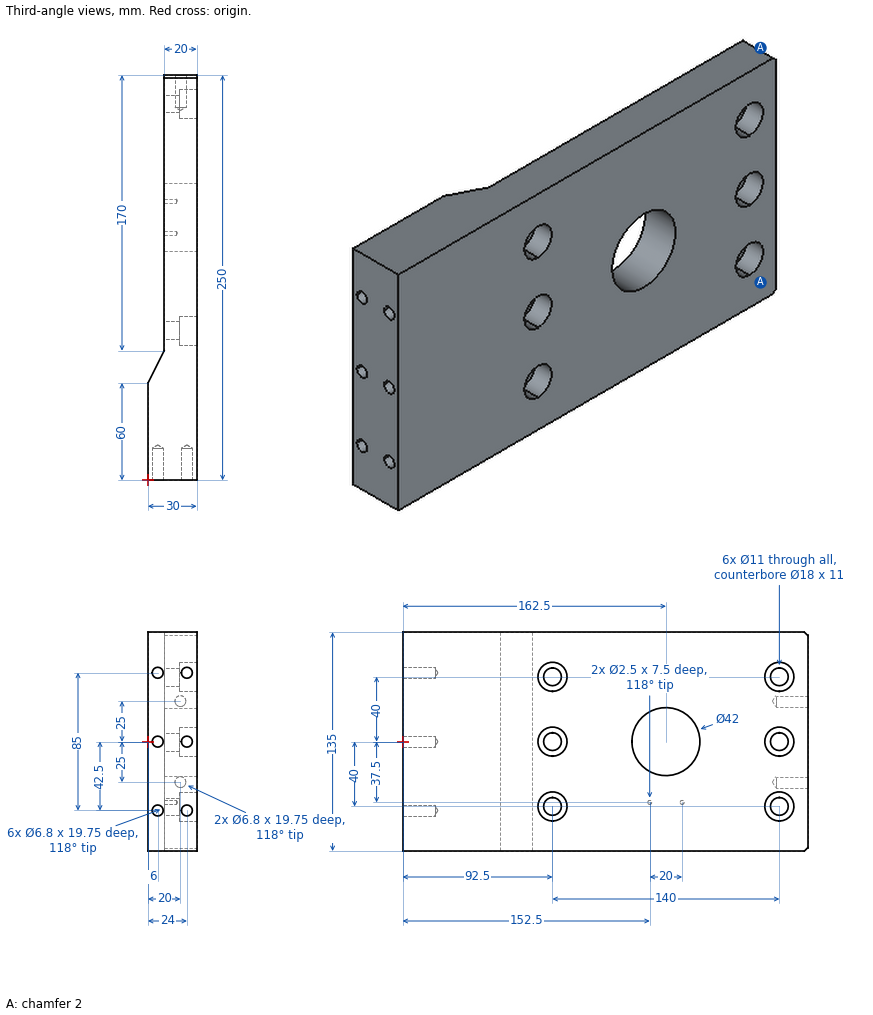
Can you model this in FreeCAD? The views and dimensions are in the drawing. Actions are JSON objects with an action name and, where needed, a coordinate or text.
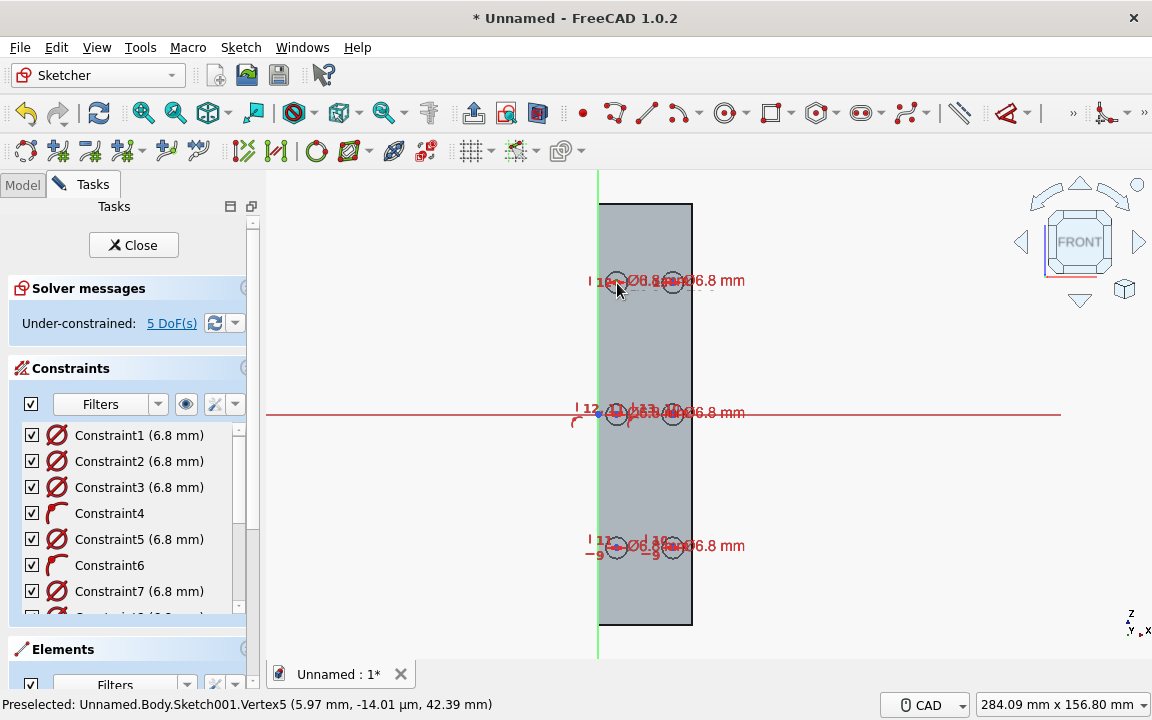
{"action": "left_click", "coordinate": [673, 283]}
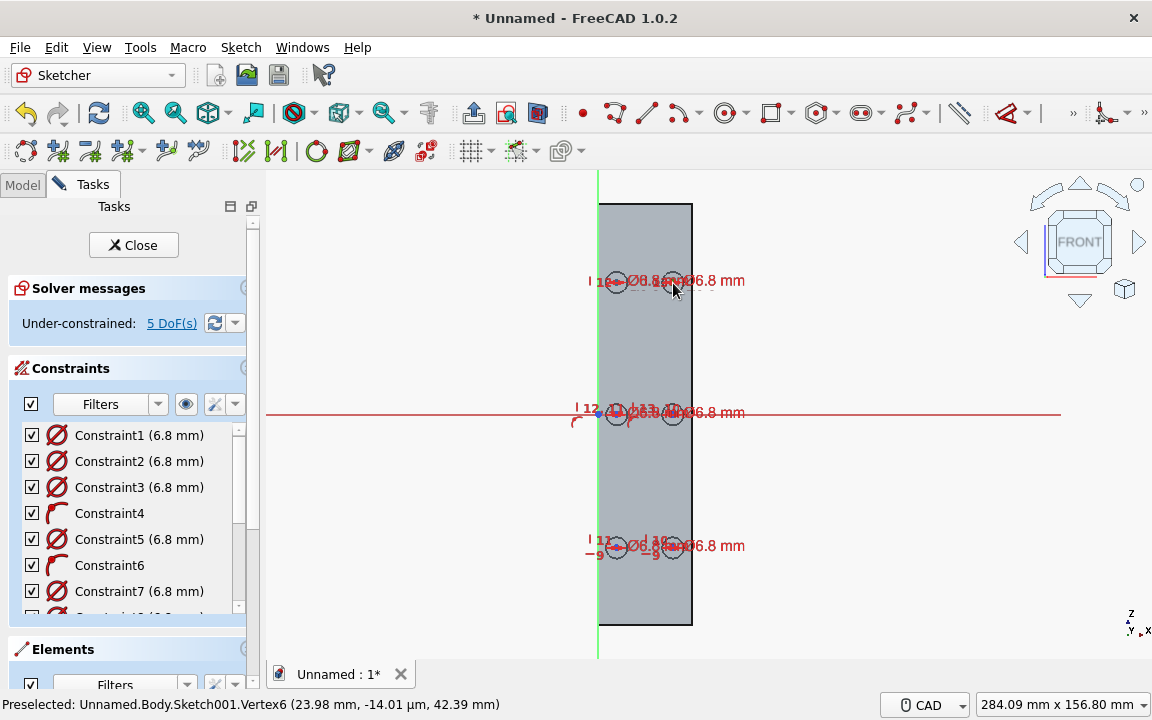
{"action": "key", "text": "h"}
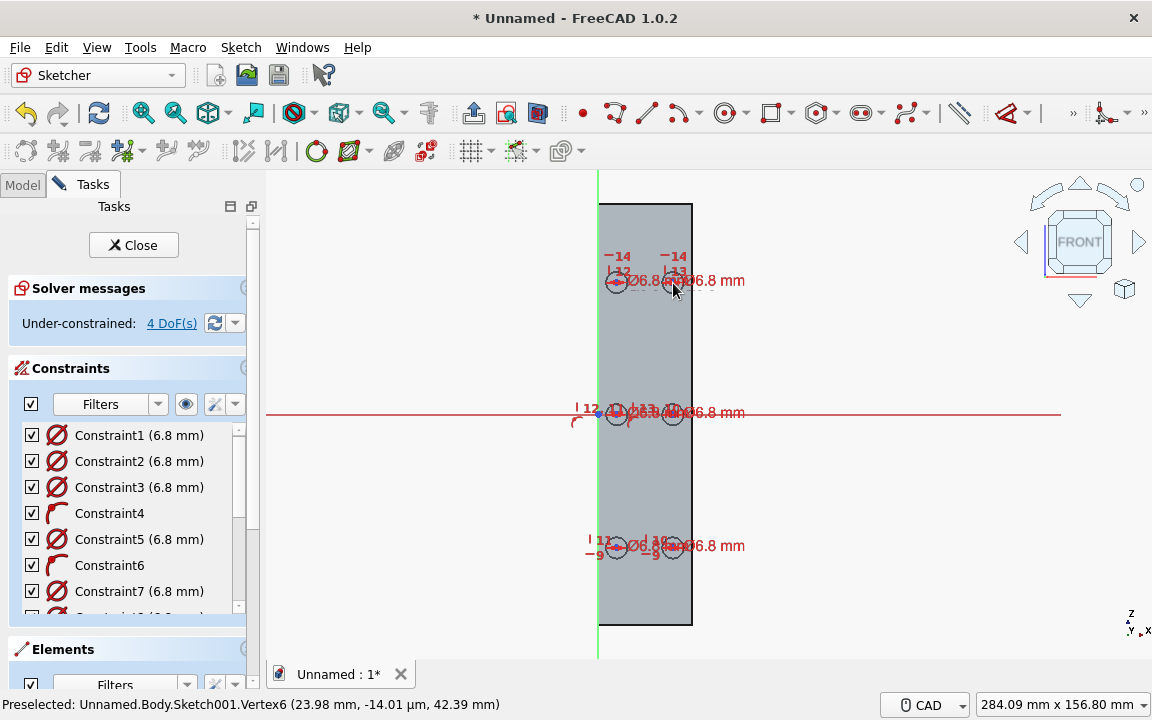
{"action": "left_click", "coordinate": [1006, 114]}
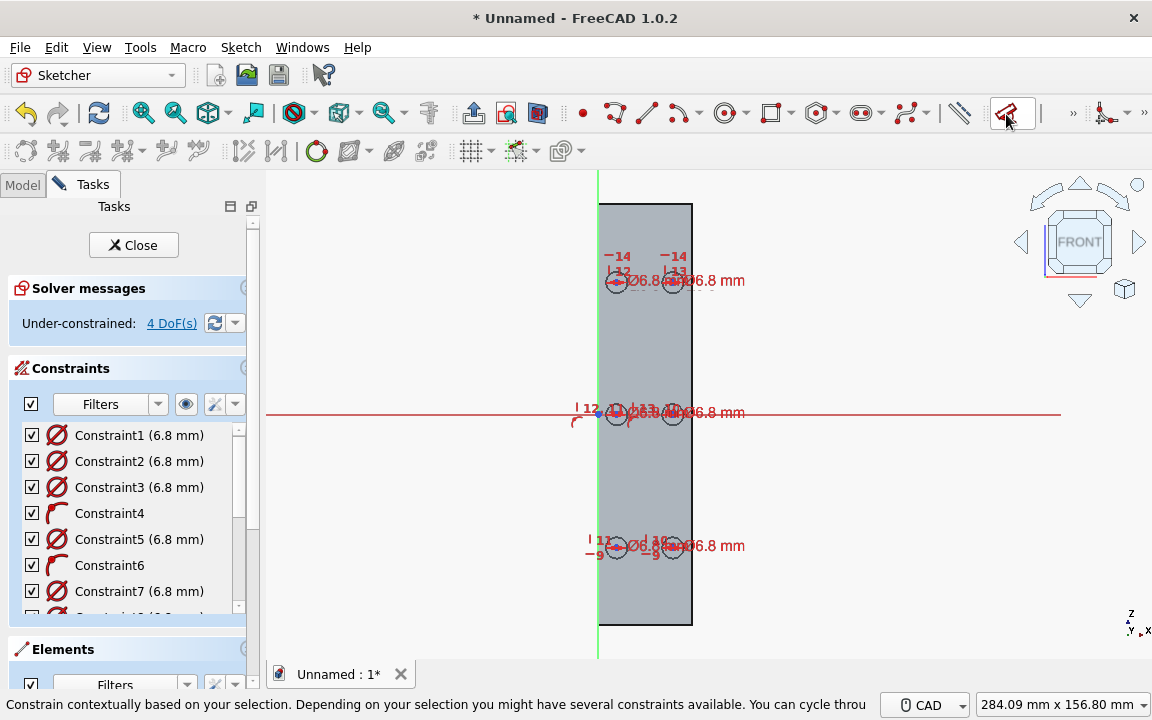
{"action": "scroll", "coordinate": [617, 548], "scroll_direction": "up", "scroll_amount": 4}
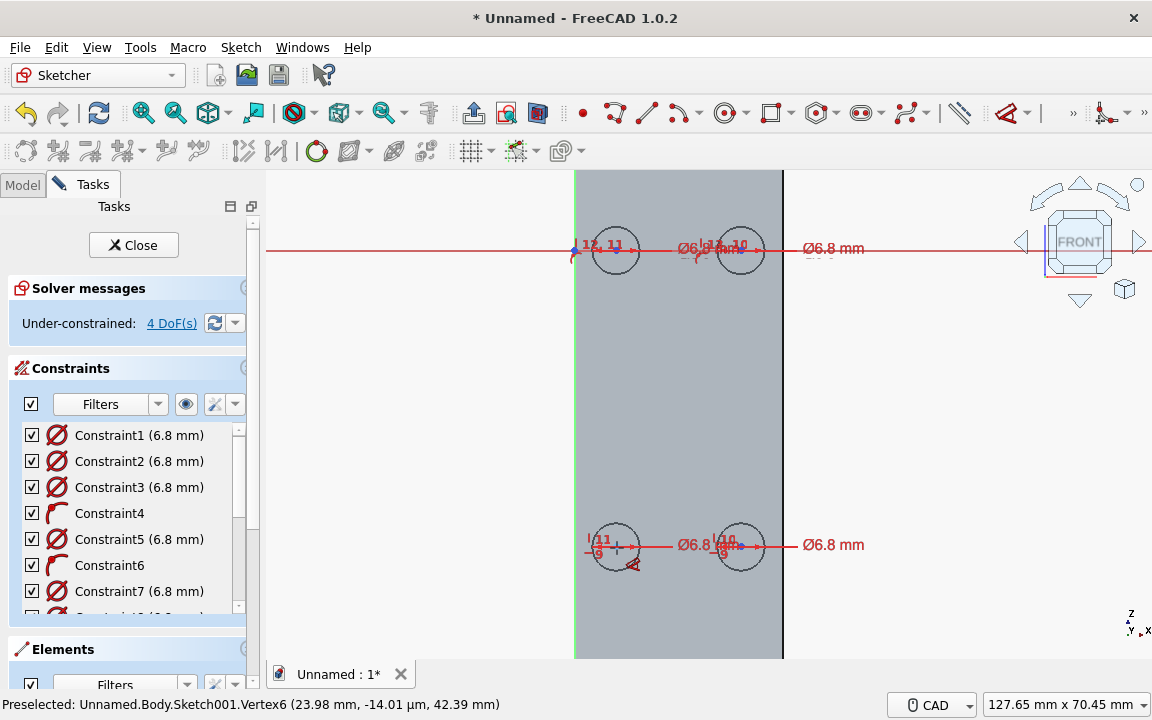
{"action": "left_click", "coordinate": [616, 547]}
{"action": "left_click", "coordinate": [595, 581]}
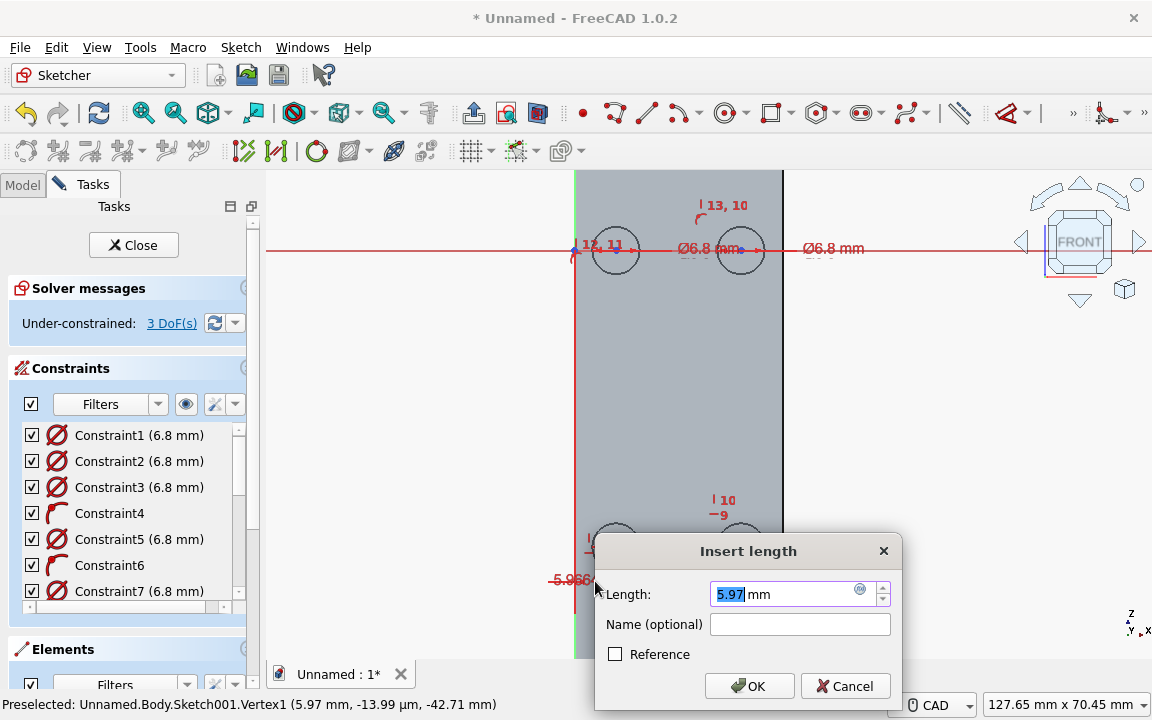
{"action": "type", "text": "6"}
{"action": "key", "text": "Return"}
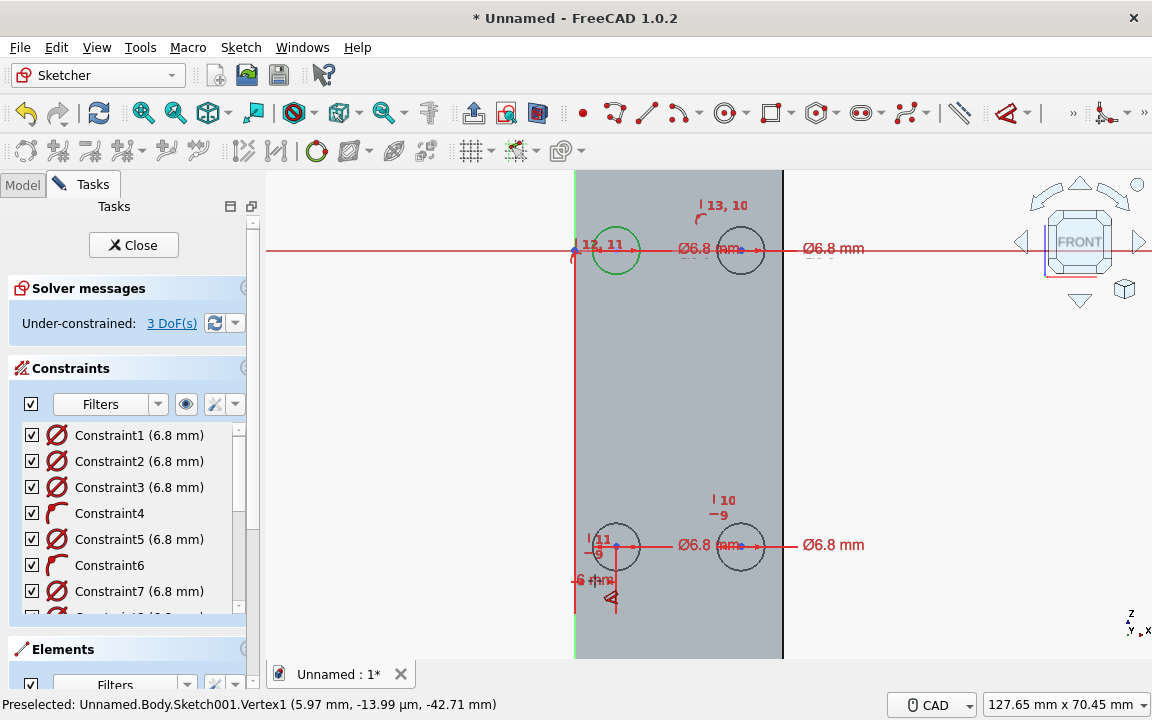
{"action": "left_click", "coordinate": [741, 547]}
{"action": "left_click", "coordinate": [696, 581]}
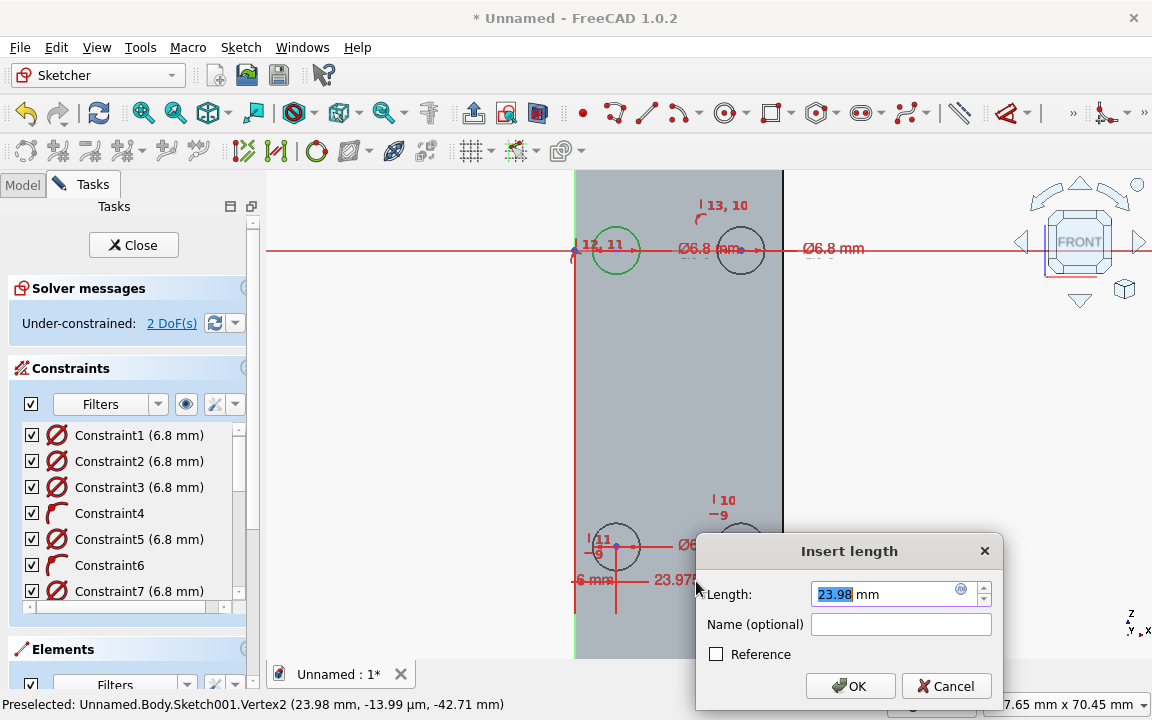
{"action": "type", "text": "24"}
{"action": "key", "text": "Return"}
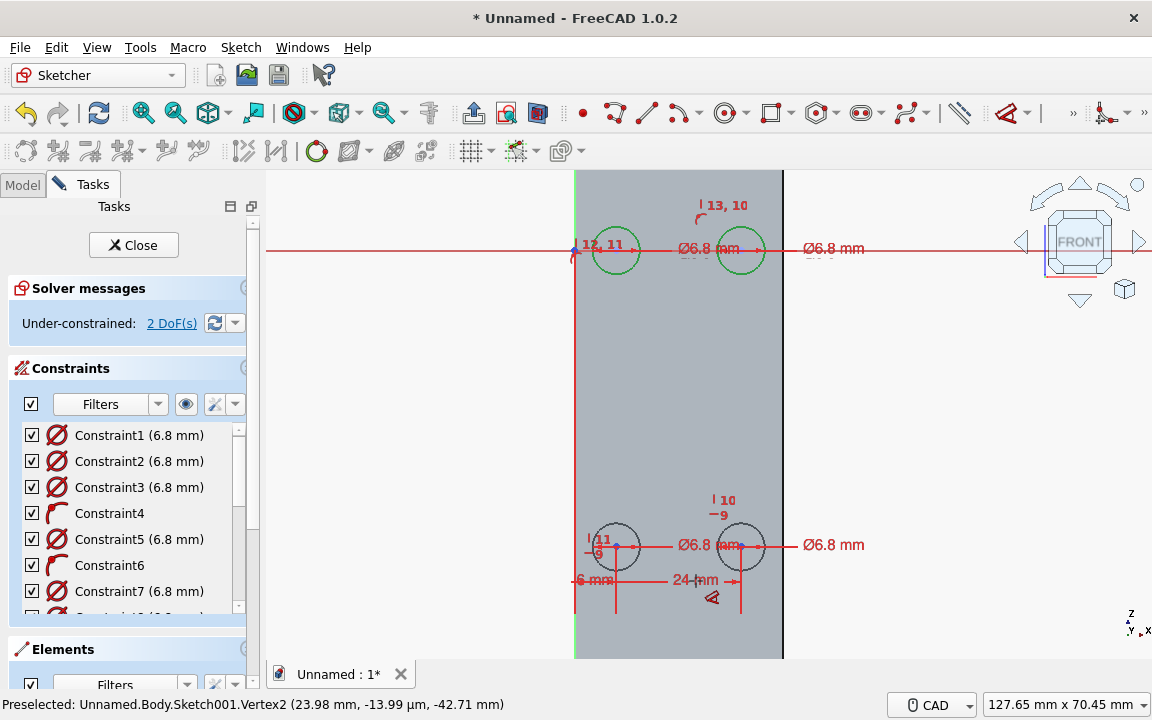
{"action": "left_click", "coordinate": [616, 547]}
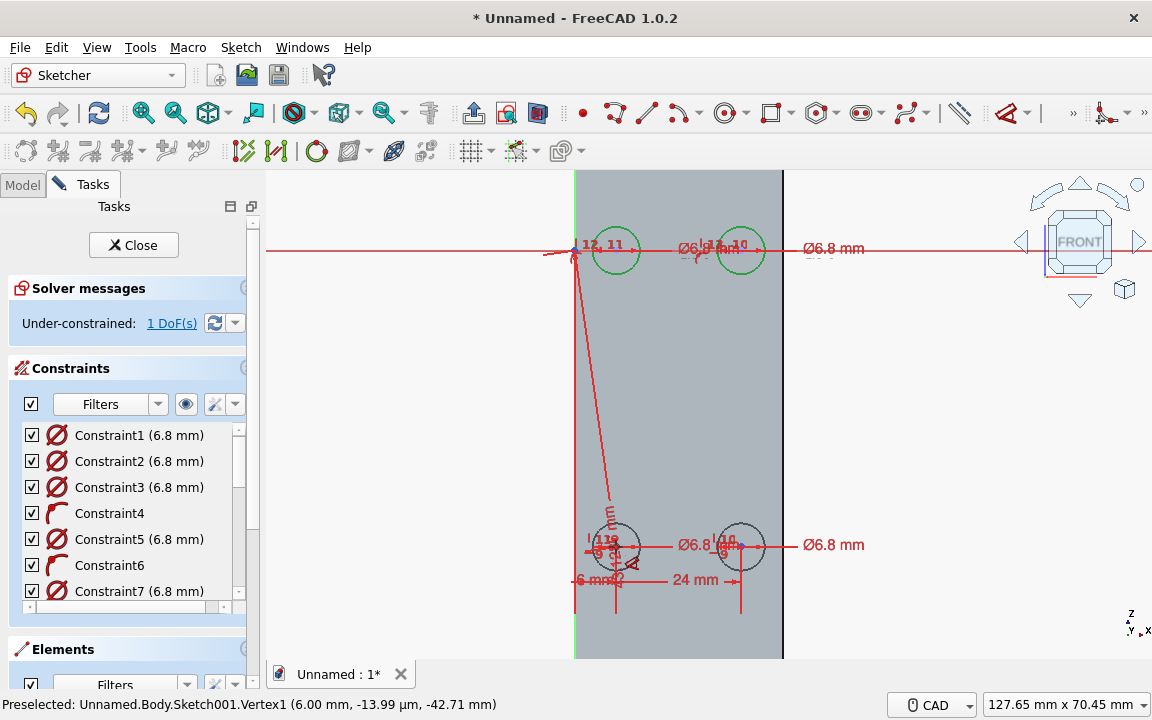
{"action": "scroll", "coordinate": [617, 548], "scroll_direction": "down", "scroll_amount": 4}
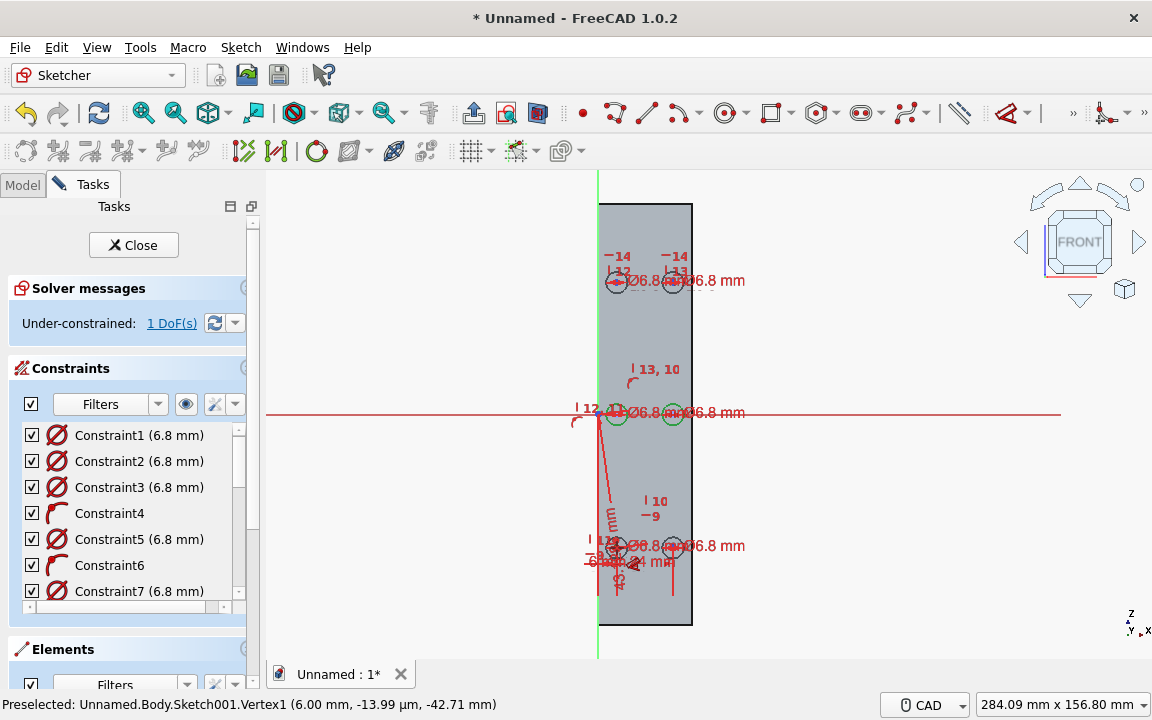
{"action": "left_click", "coordinate": [617, 283]}
{"action": "left_click", "coordinate": [583, 354]}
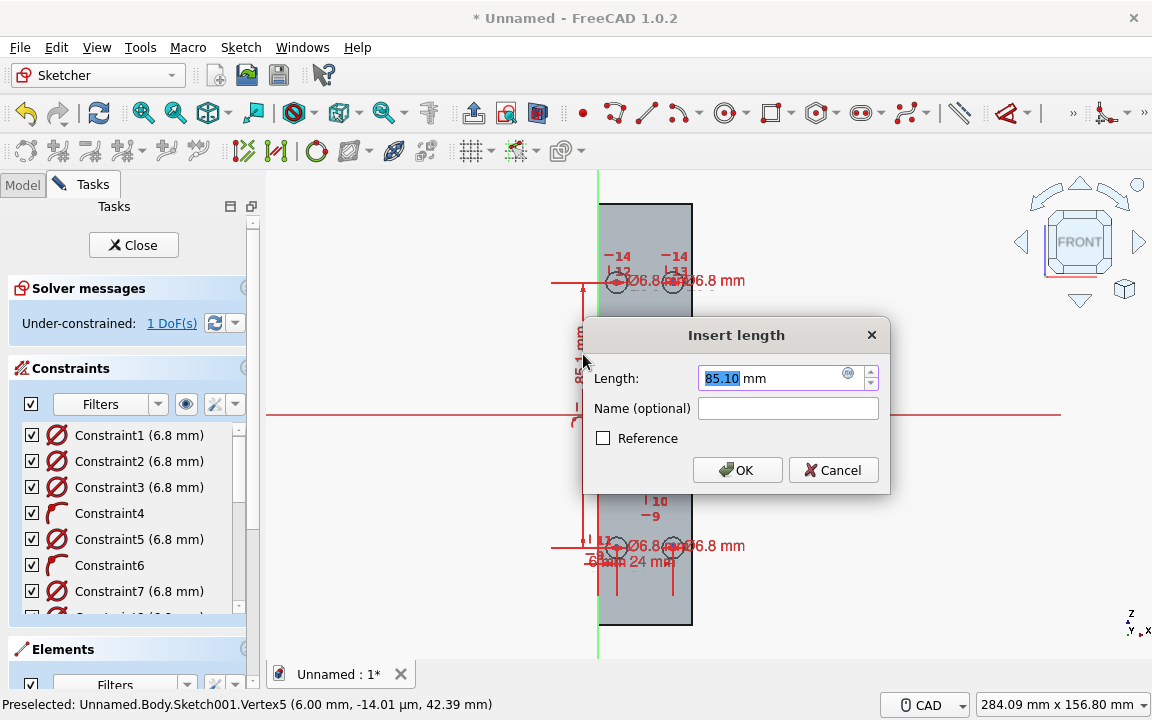
{"action": "type", "text": "85"}
{"action": "key", "text": "Return"}